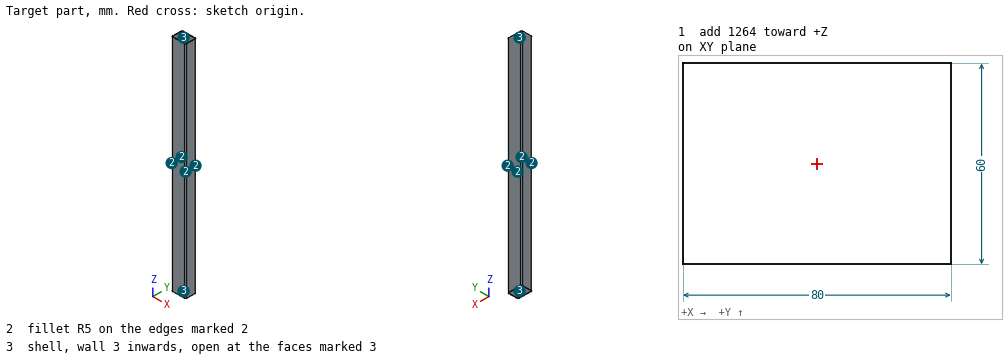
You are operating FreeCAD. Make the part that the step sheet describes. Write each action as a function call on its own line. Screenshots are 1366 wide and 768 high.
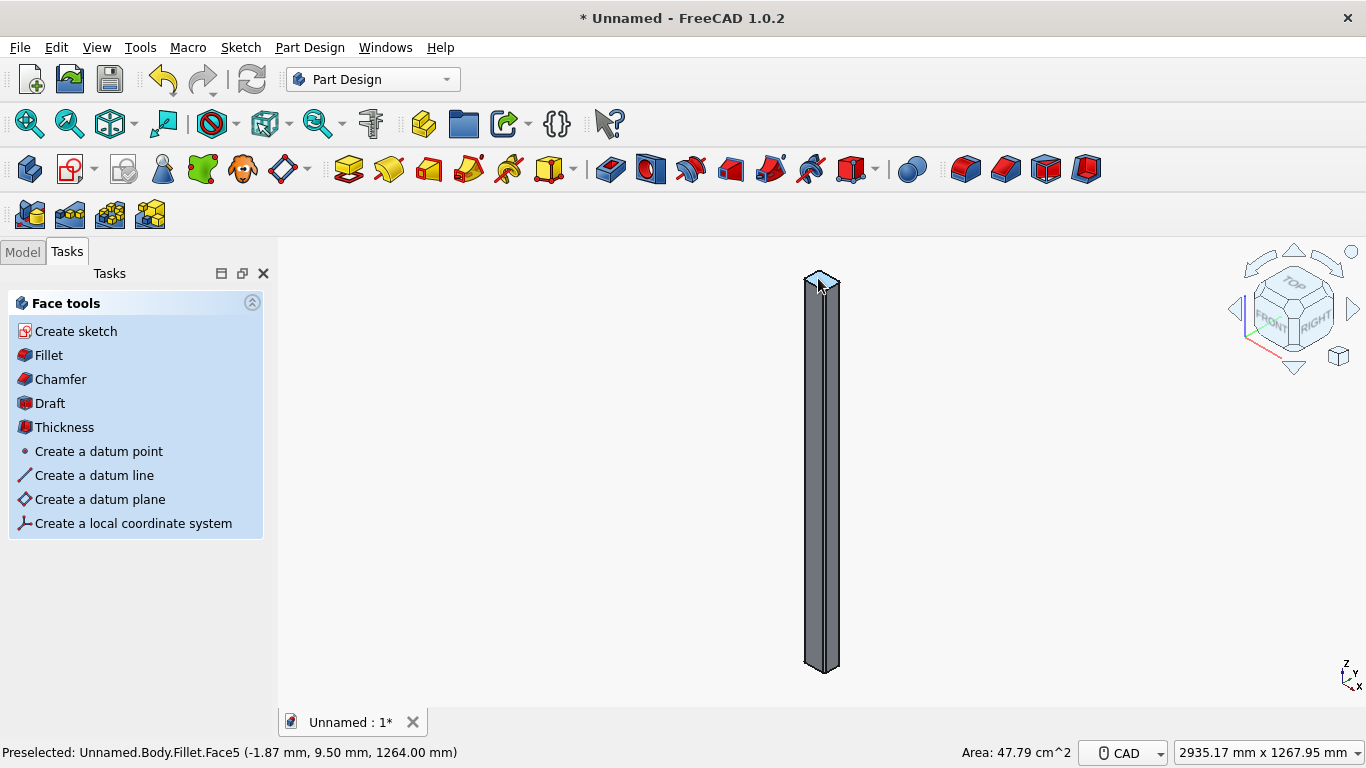
key(2)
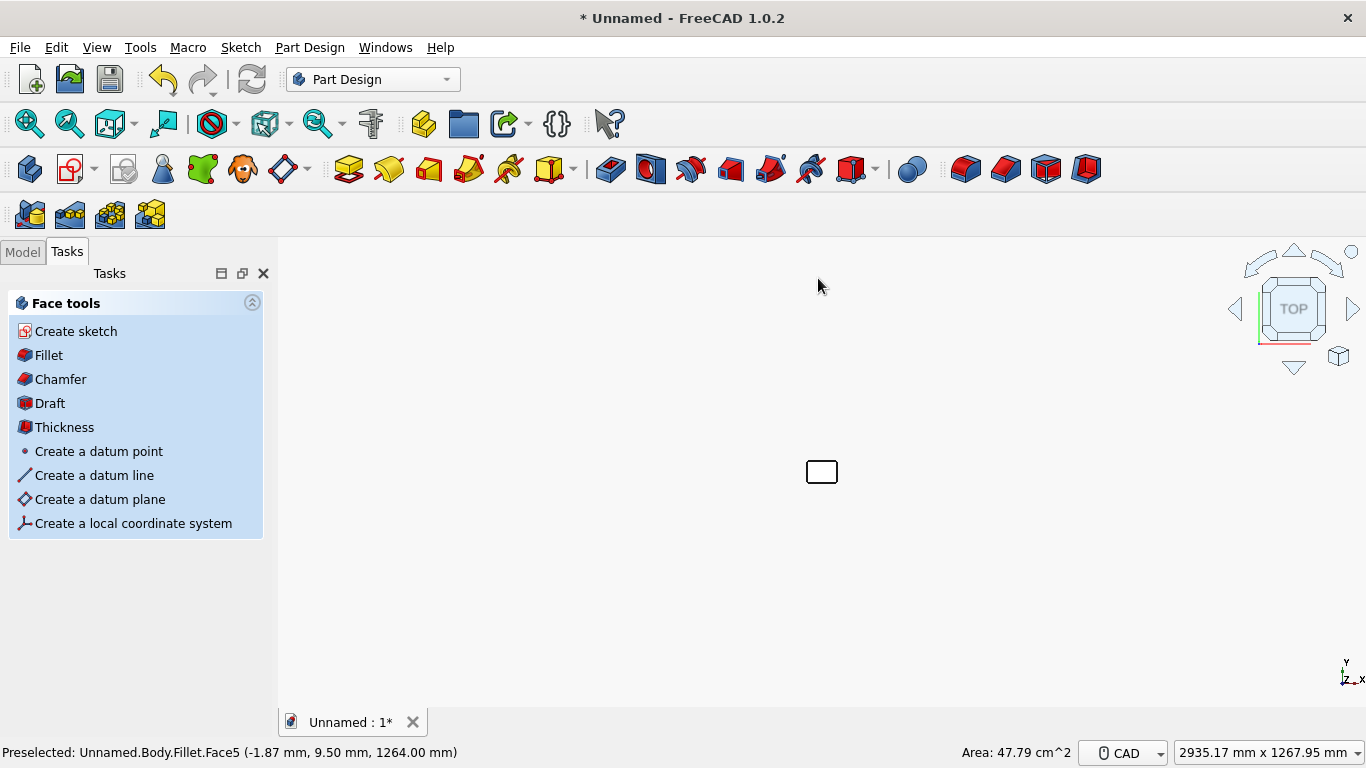
key(v)
key(f)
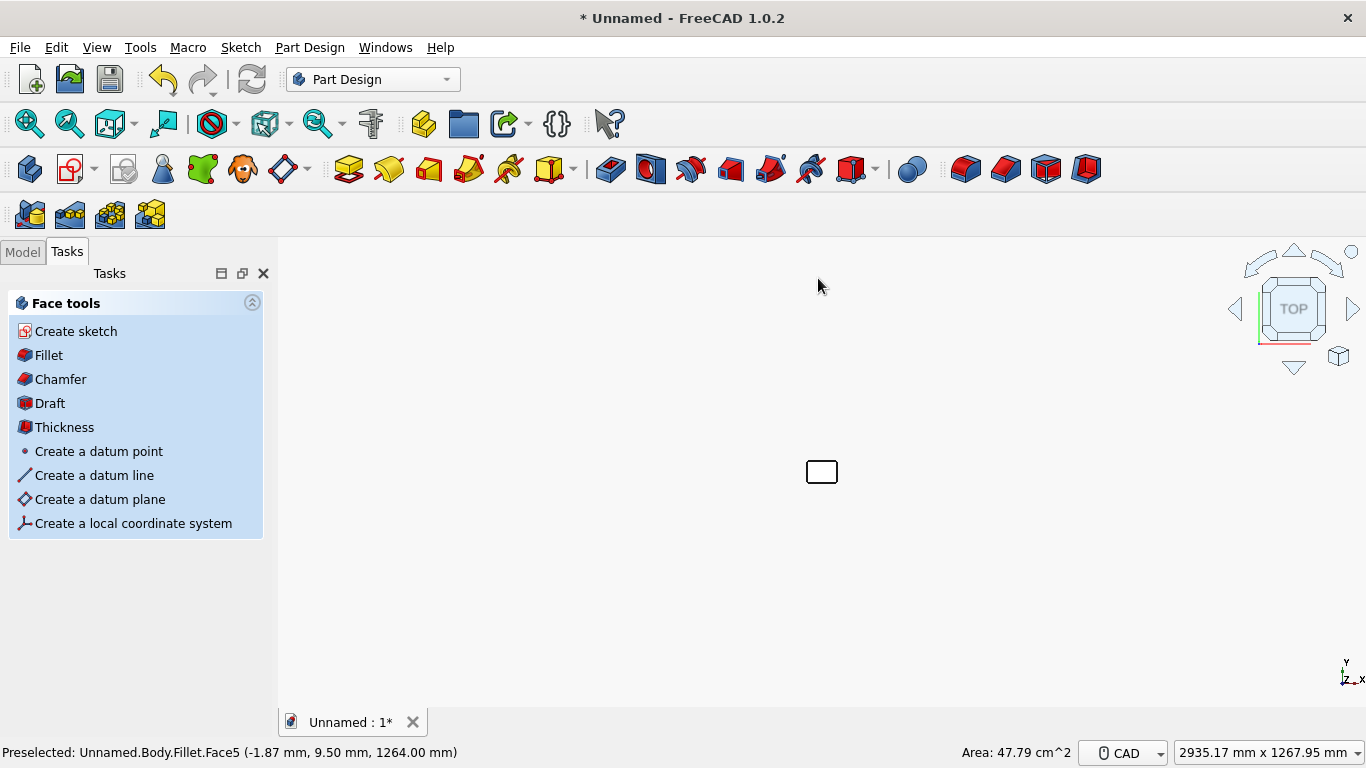
key(1)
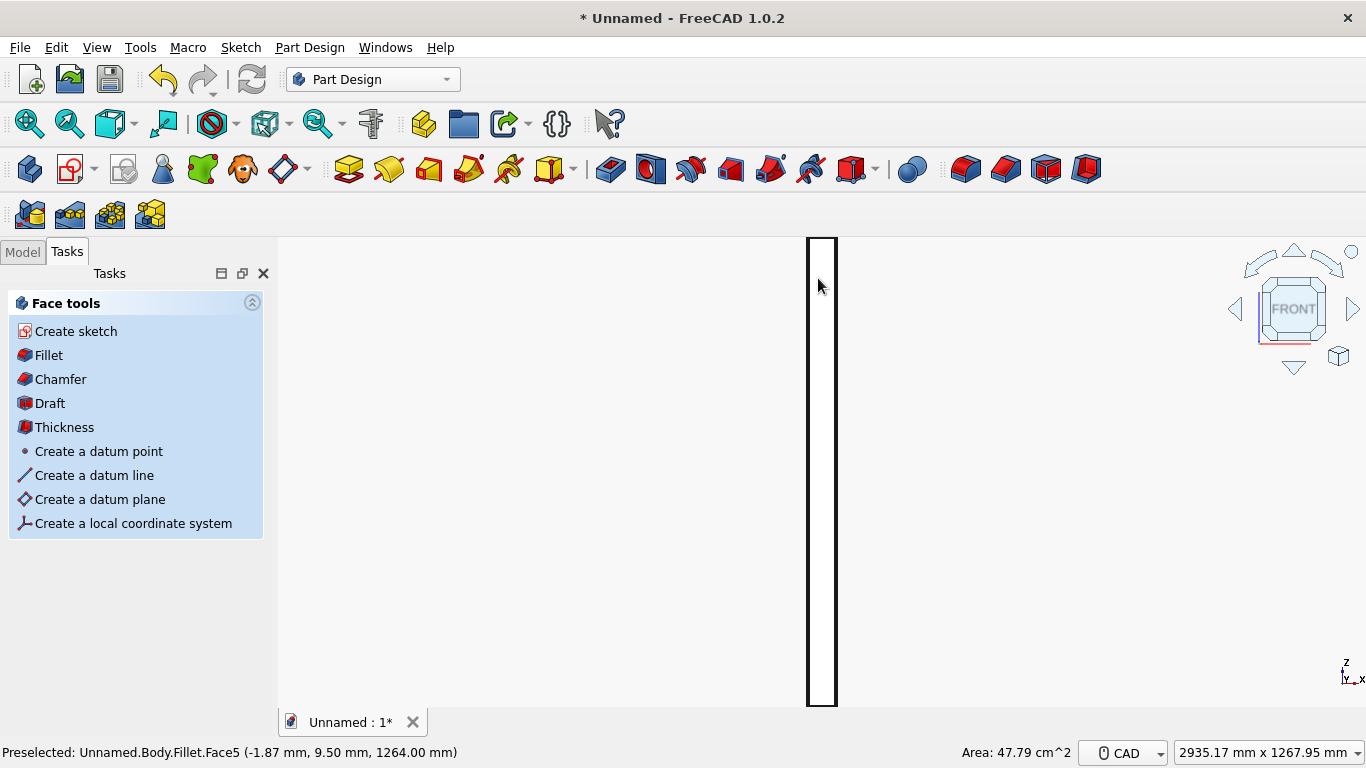
key(3)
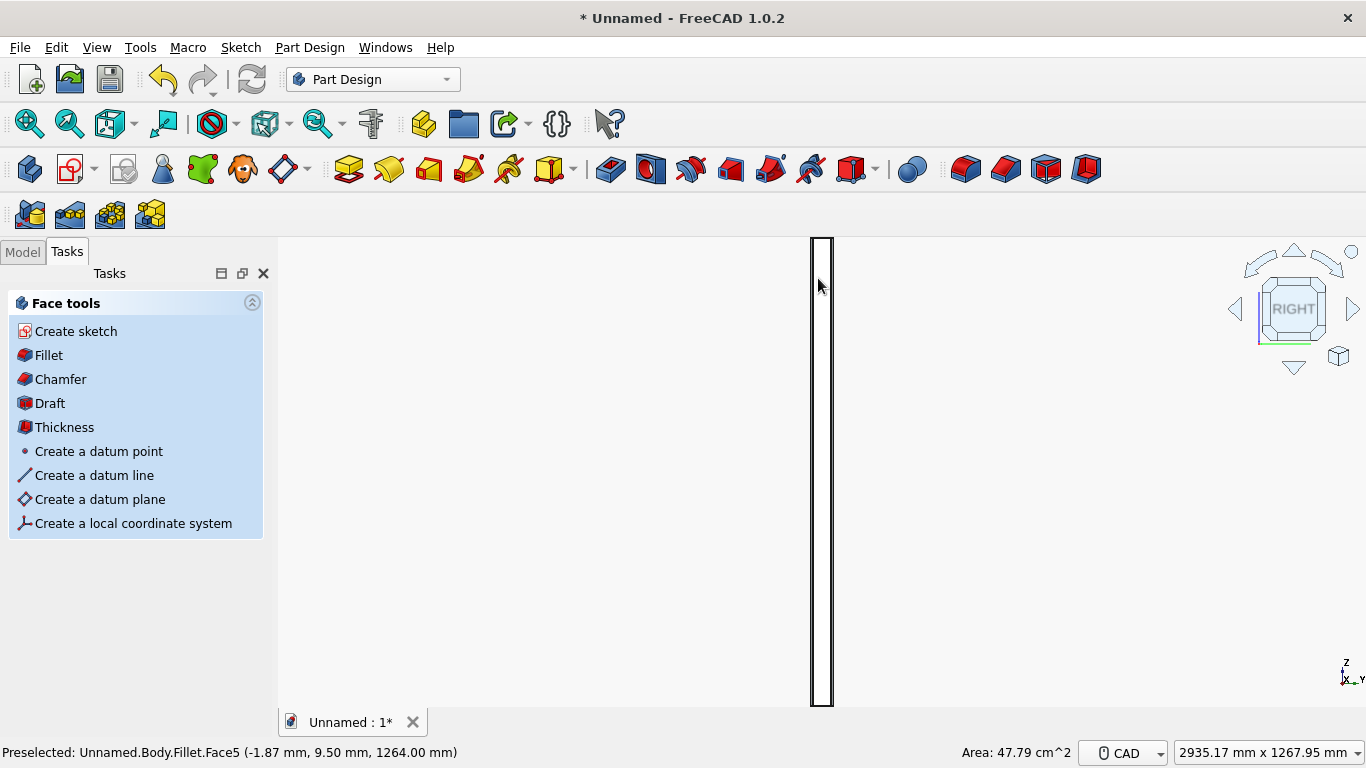
key(5)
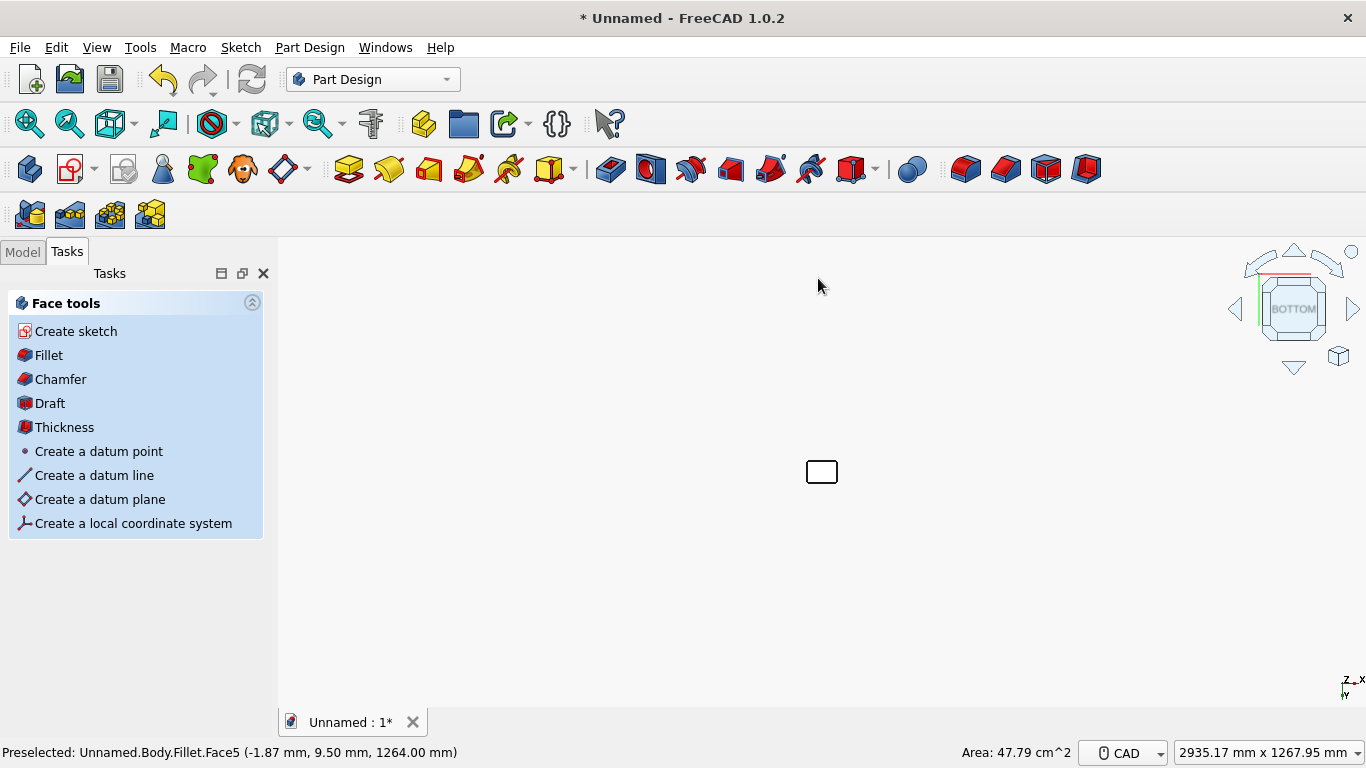
key(v)
key(f)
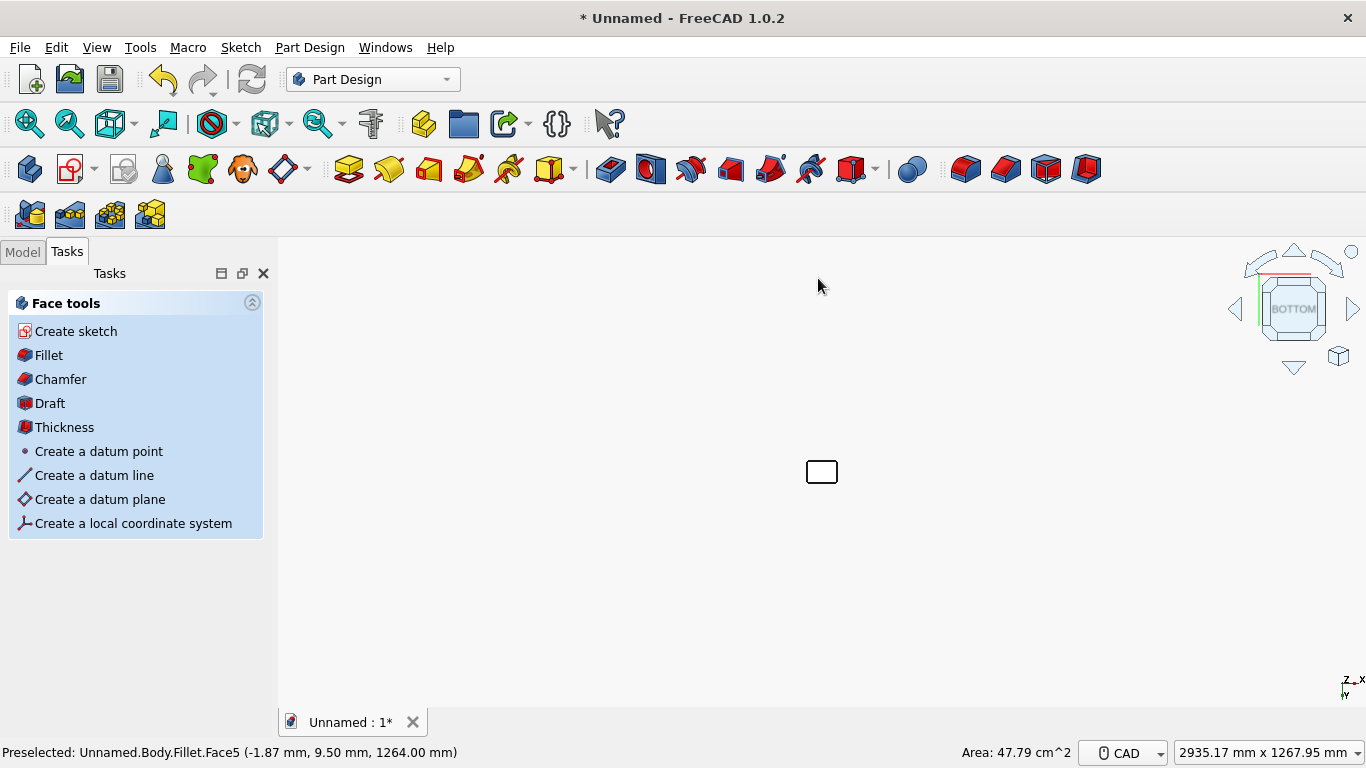
click(822, 471, ctrl)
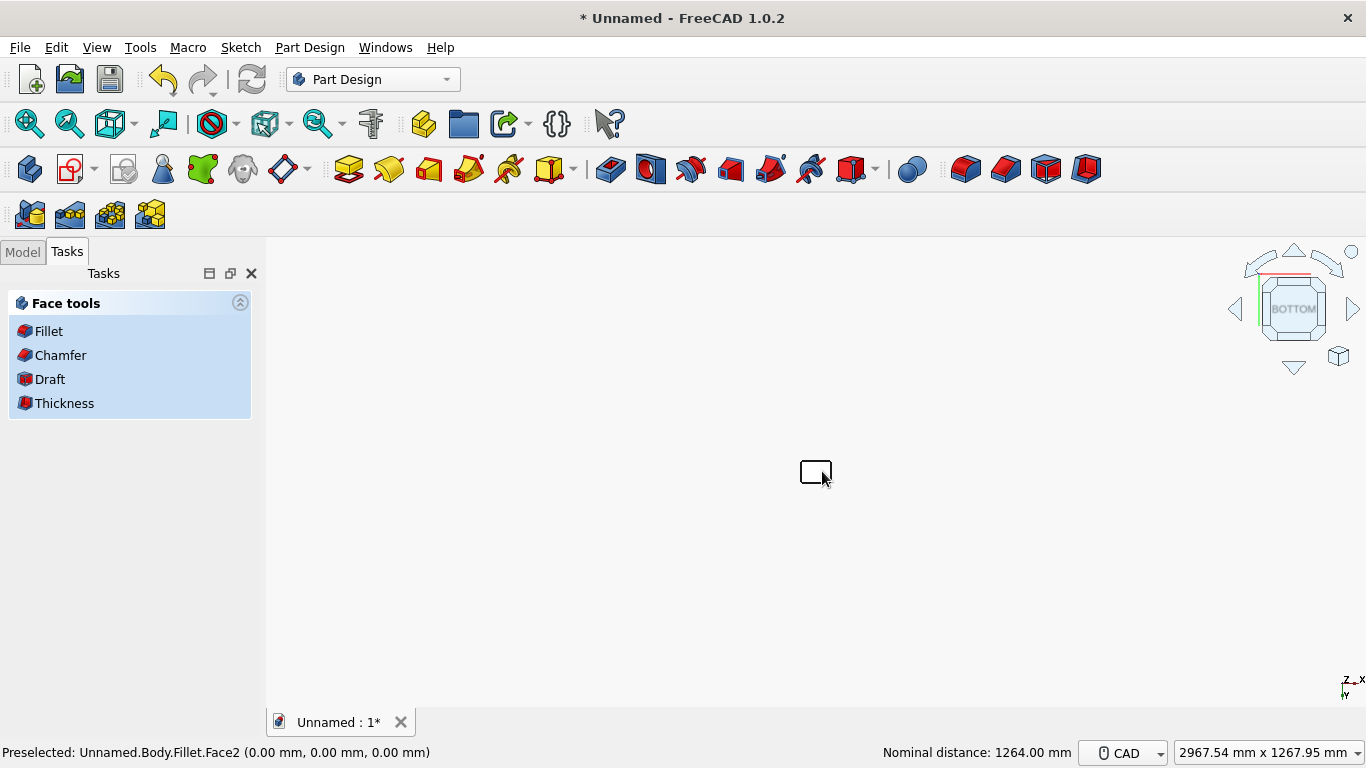
click(1086, 170)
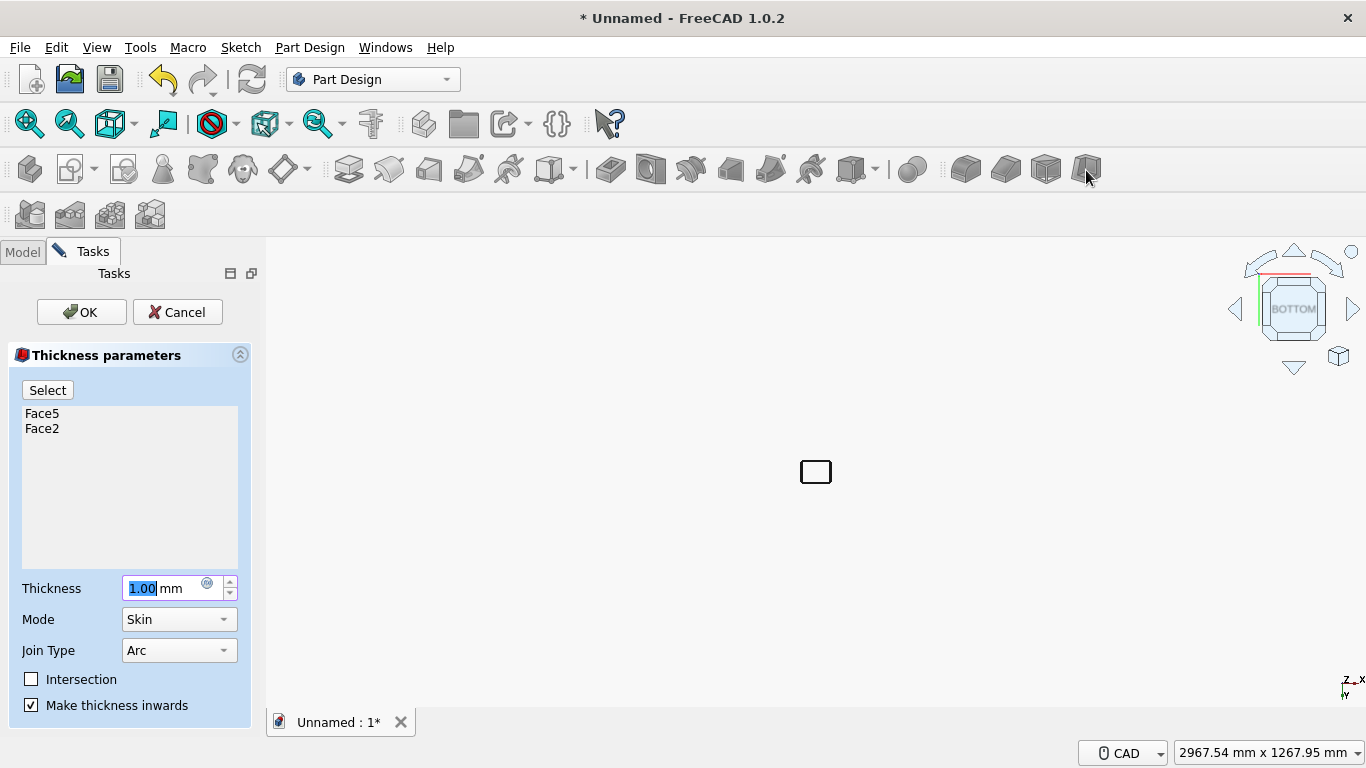
text(3)
key(Tab)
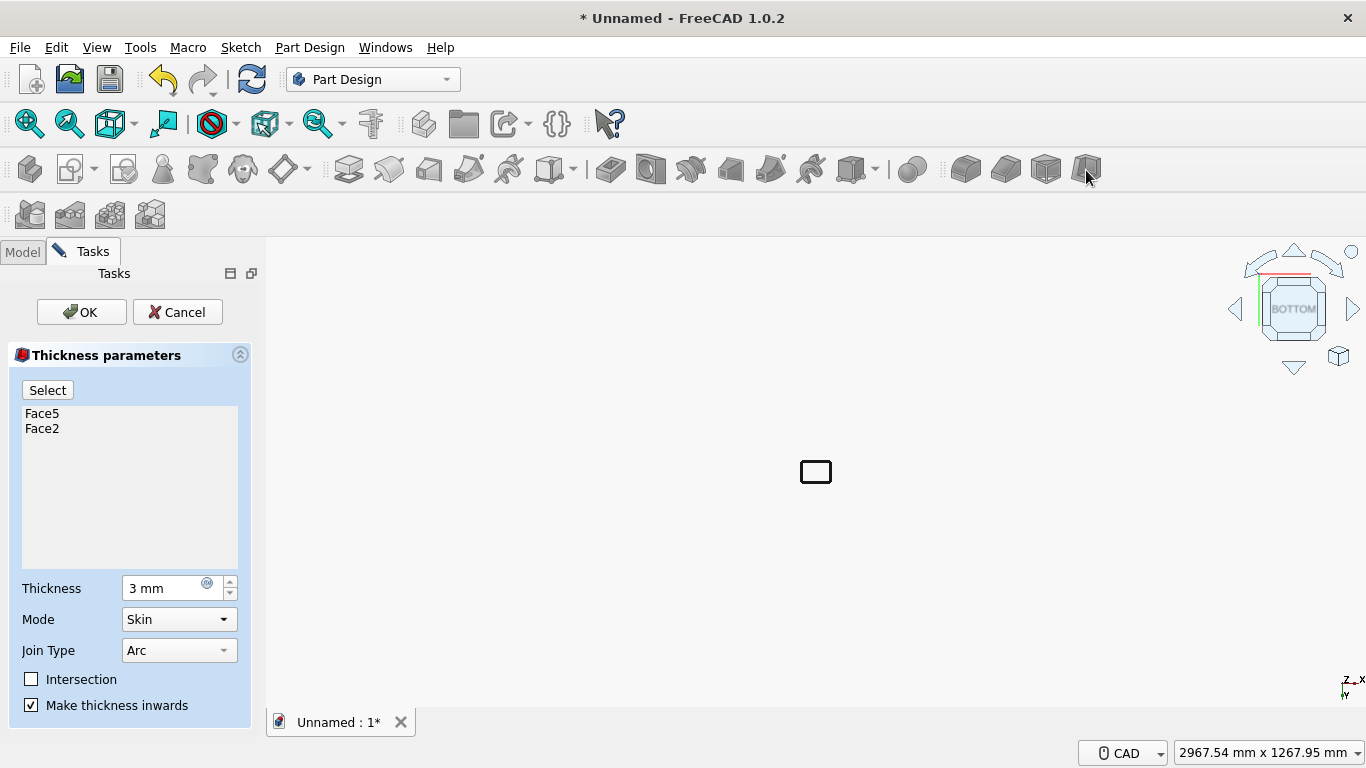
click(180, 650)